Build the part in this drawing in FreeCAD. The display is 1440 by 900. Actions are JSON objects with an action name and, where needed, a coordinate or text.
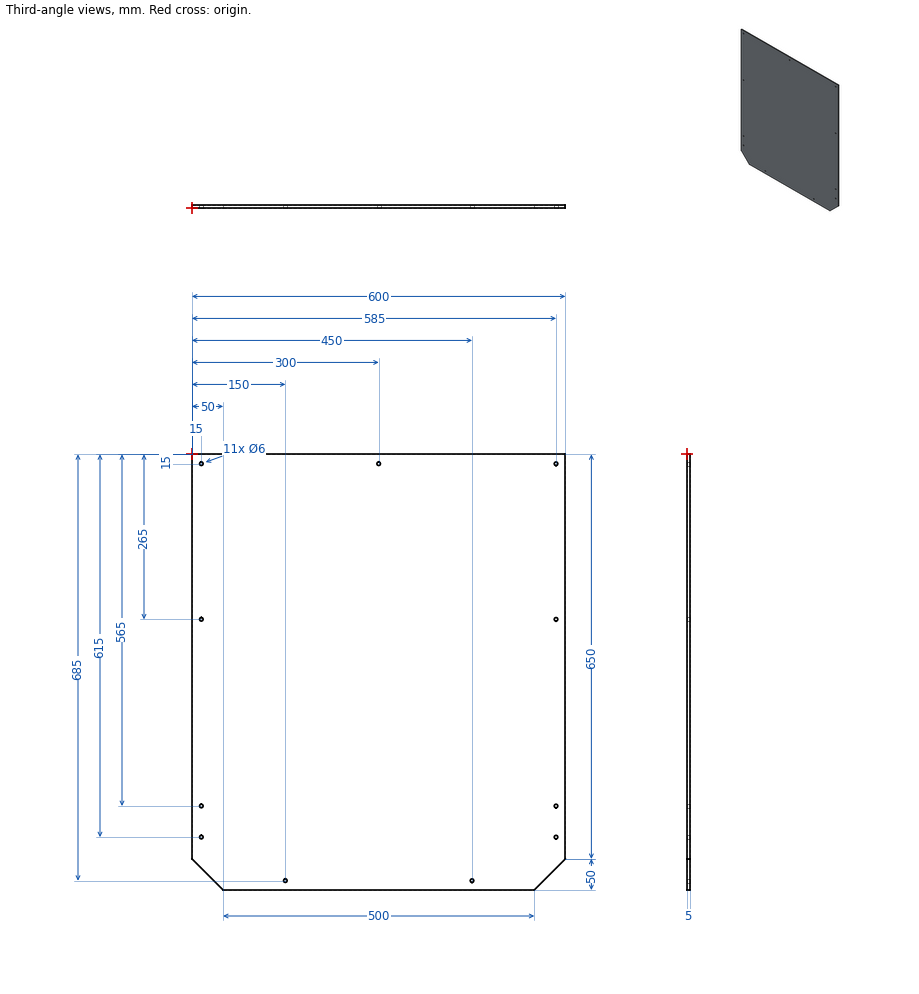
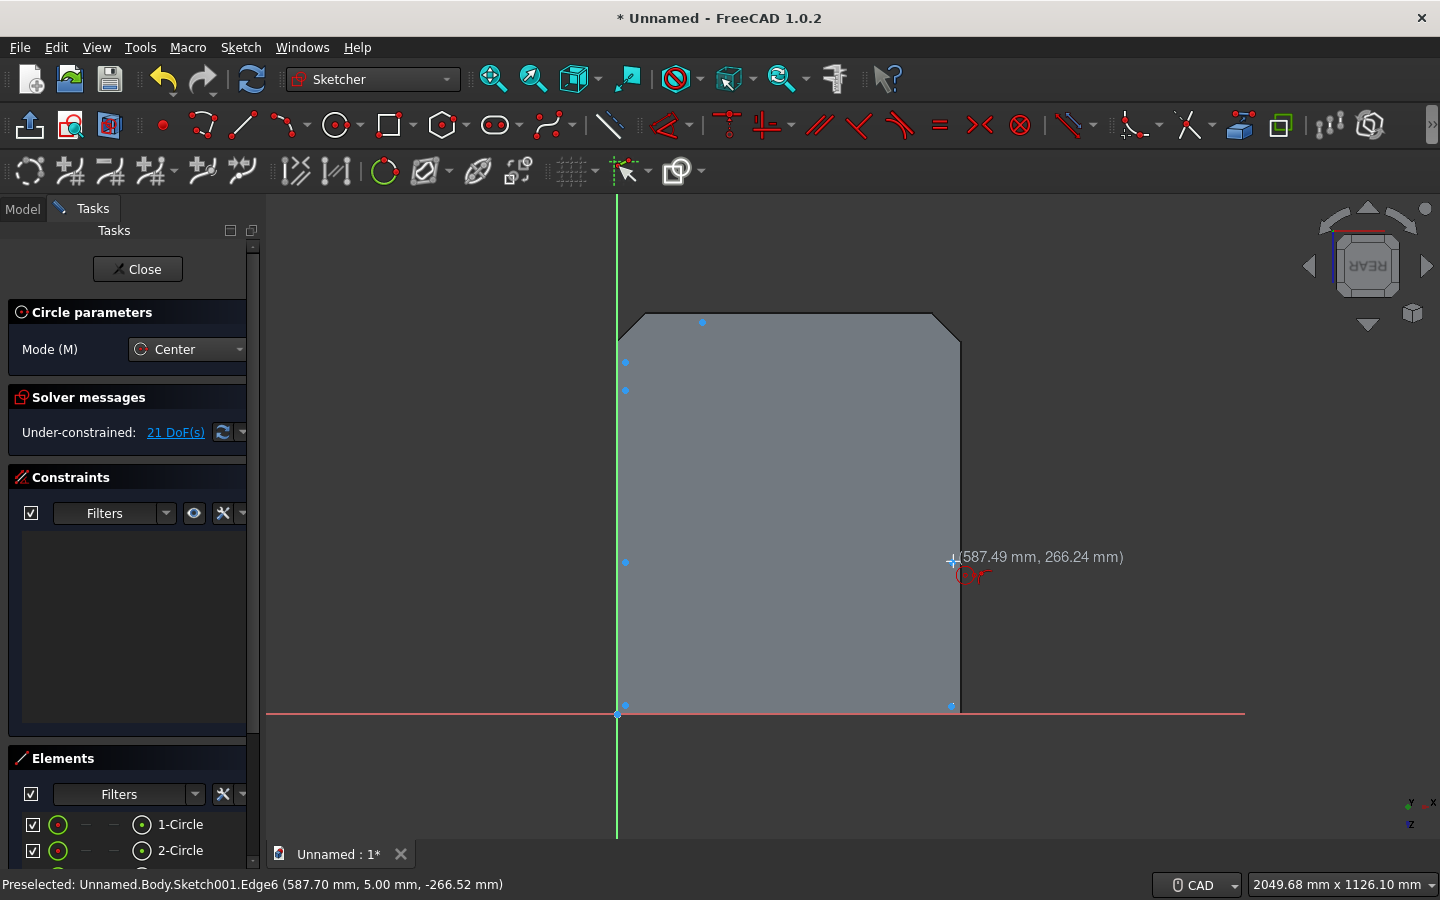
{"action": "scroll", "coordinate": [952, 390], "scroll_direction": "up", "scroll_amount": 13}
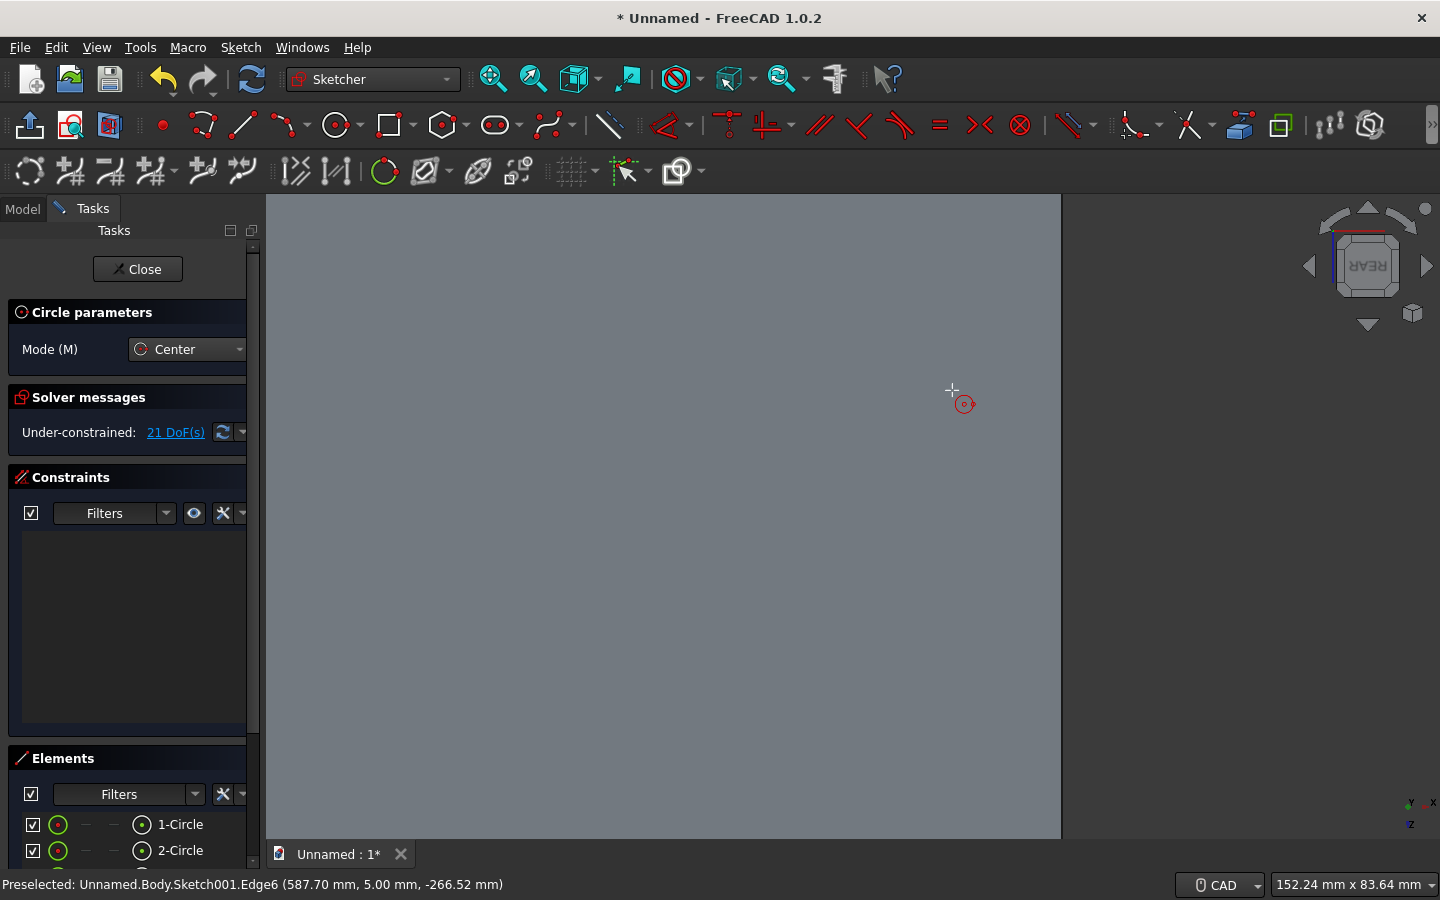
{"action": "scroll", "coordinate": [952, 390], "scroll_direction": "down", "scroll_amount": 13}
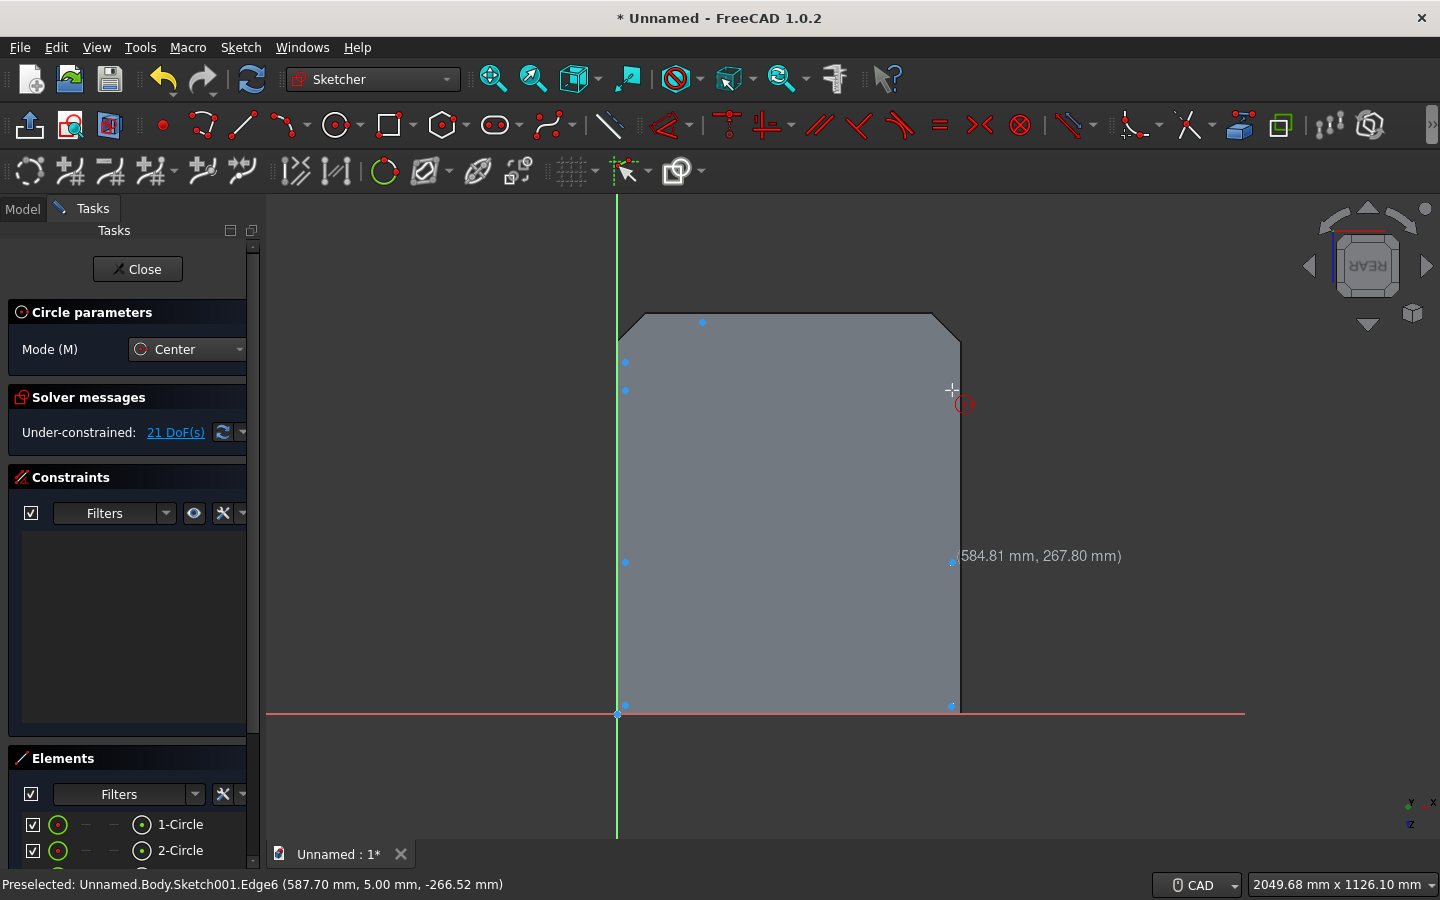
{"action": "left_click", "coordinate": [952, 390]}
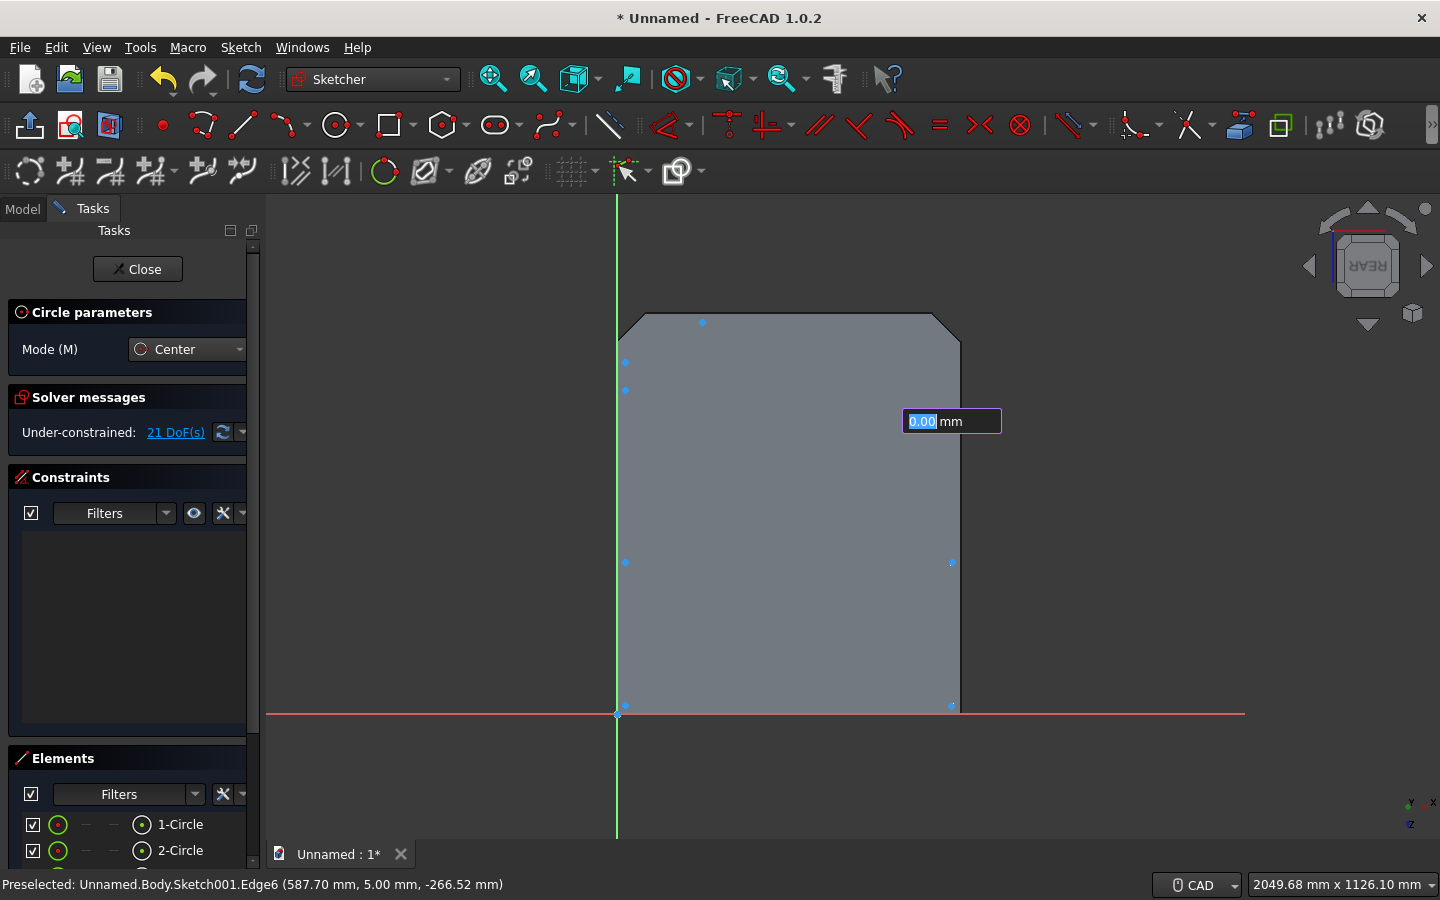
{"action": "scroll", "coordinate": [953, 389], "scroll_direction": "up", "scroll_amount": 12}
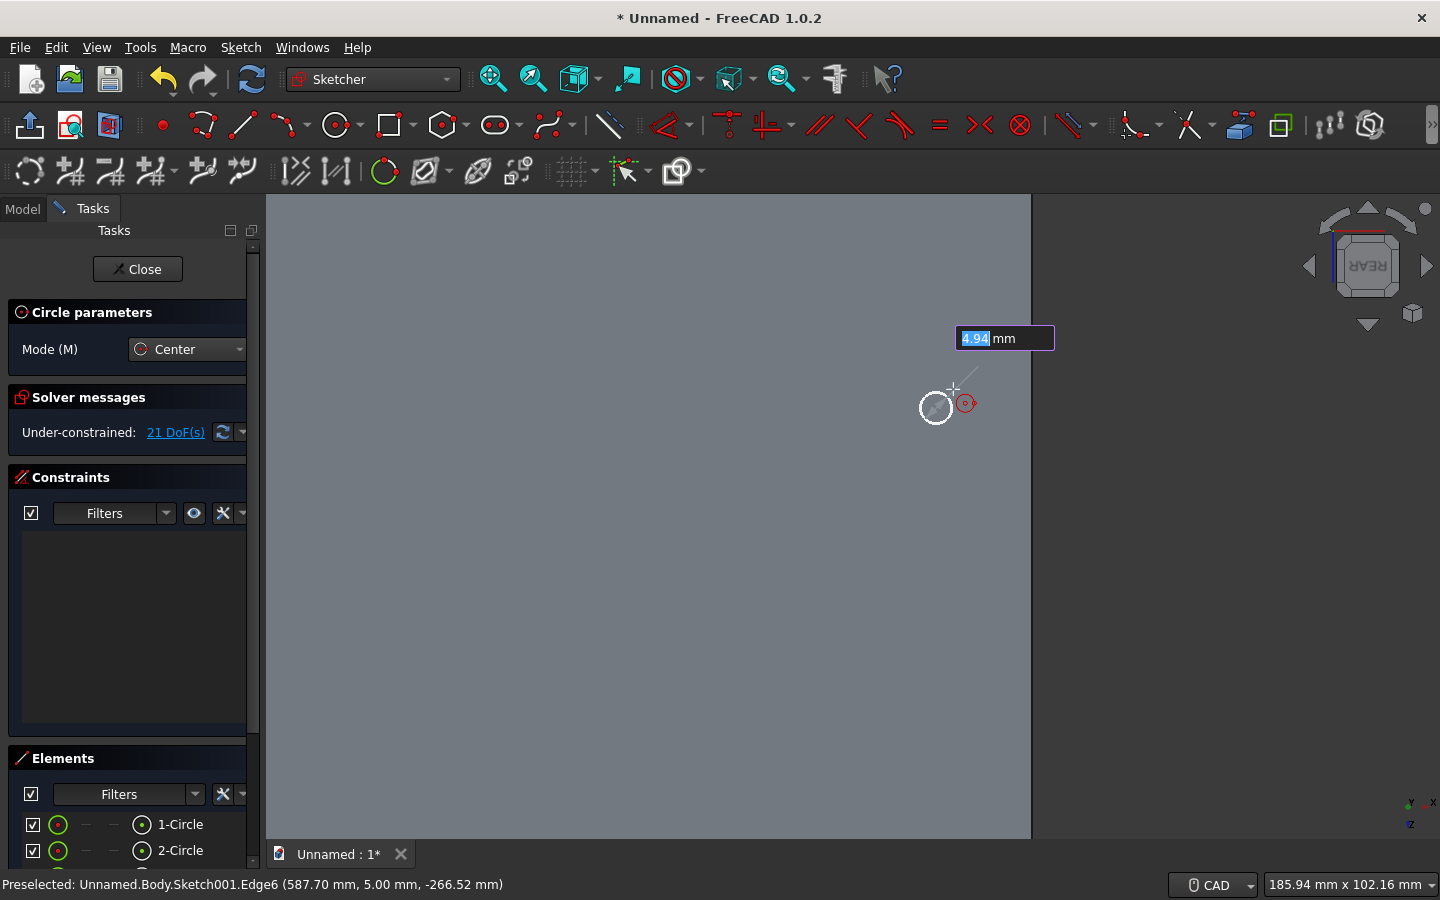
{"action": "left_click", "coordinate": [951, 389]}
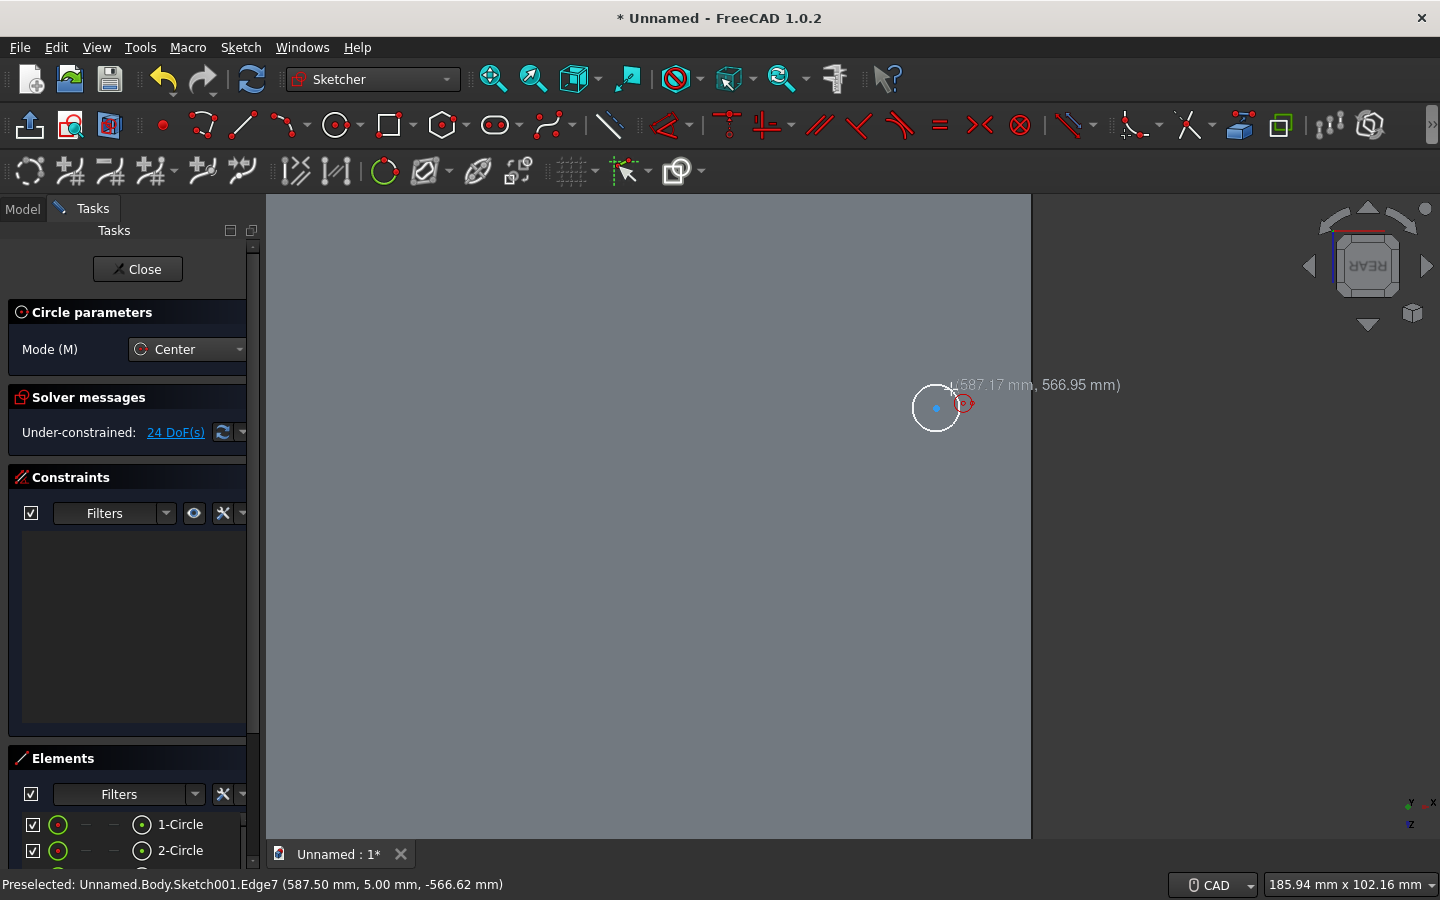
{"action": "scroll", "coordinate": [953, 389], "scroll_direction": "down", "scroll_amount": 12}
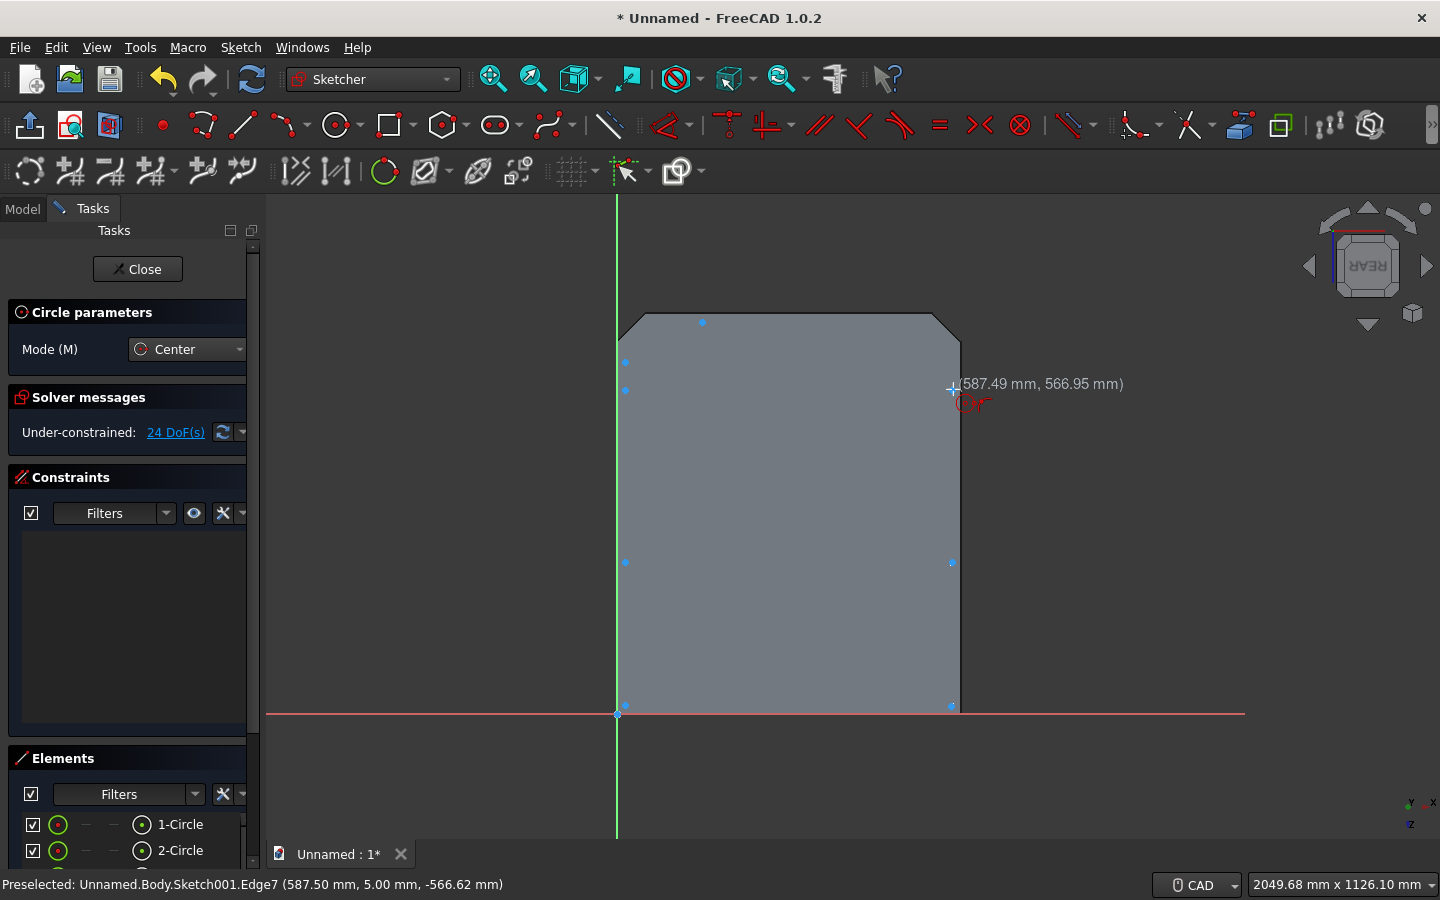
{"action": "scroll", "coordinate": [952, 362], "scroll_direction": "up", "scroll_amount": 13}